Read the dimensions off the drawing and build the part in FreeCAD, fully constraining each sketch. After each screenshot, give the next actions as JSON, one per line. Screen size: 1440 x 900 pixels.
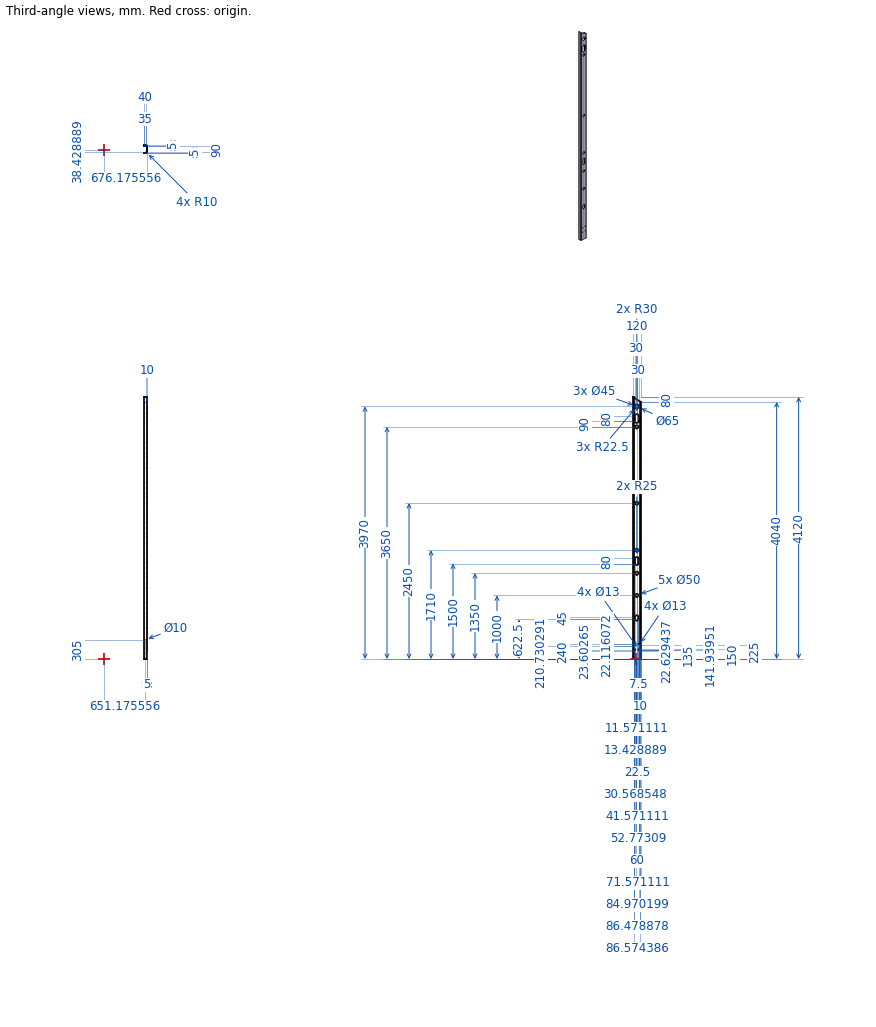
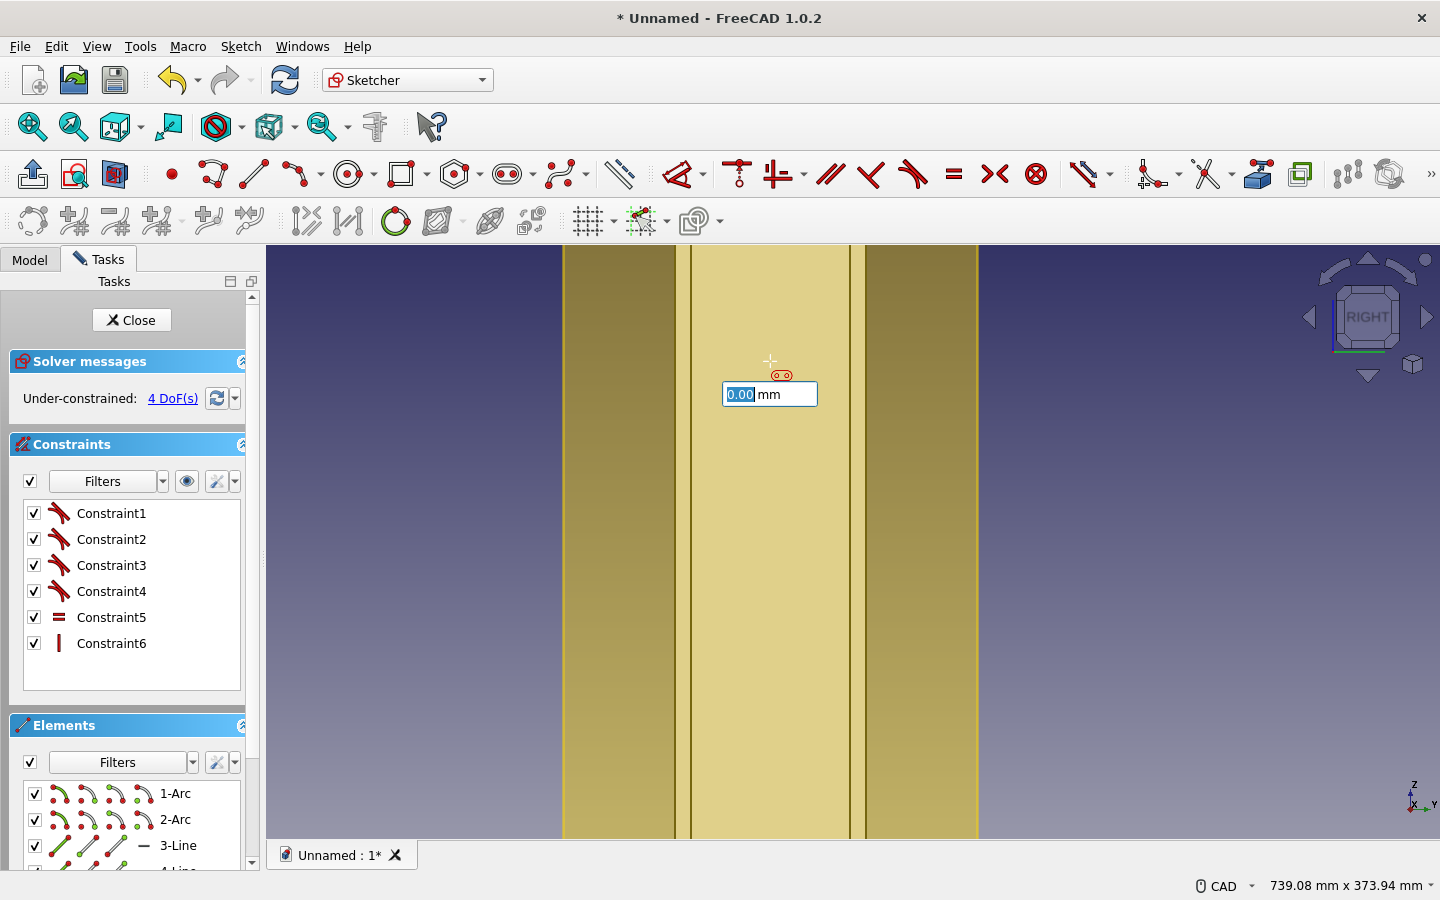
{"action": "scroll", "coordinate": [785, 366], "scroll_direction": "down", "scroll_amount": 14}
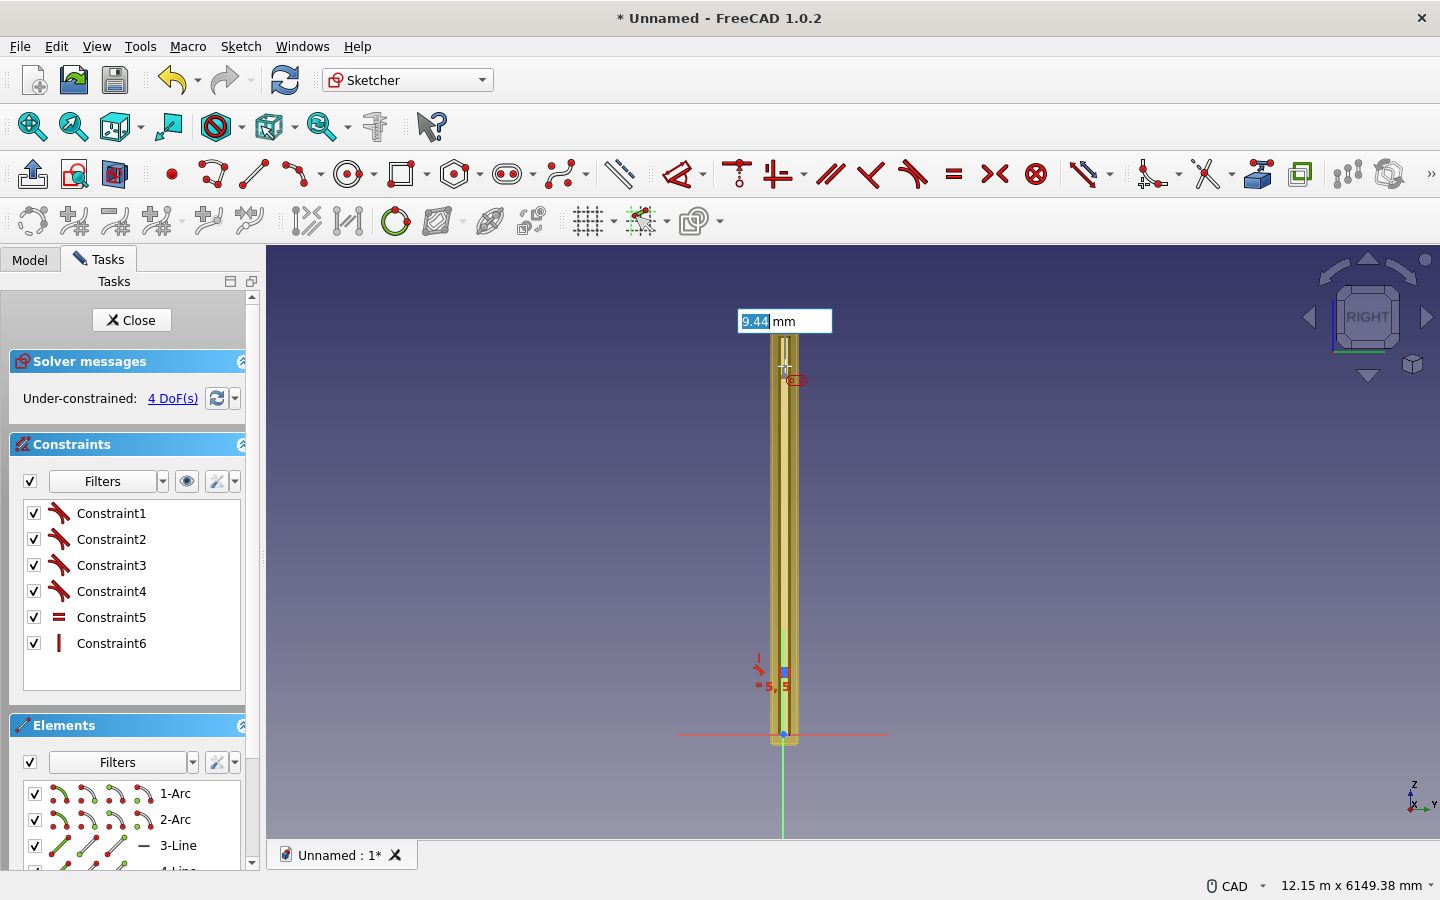
{"action": "scroll", "coordinate": [787, 370], "scroll_direction": "up", "scroll_amount": 9}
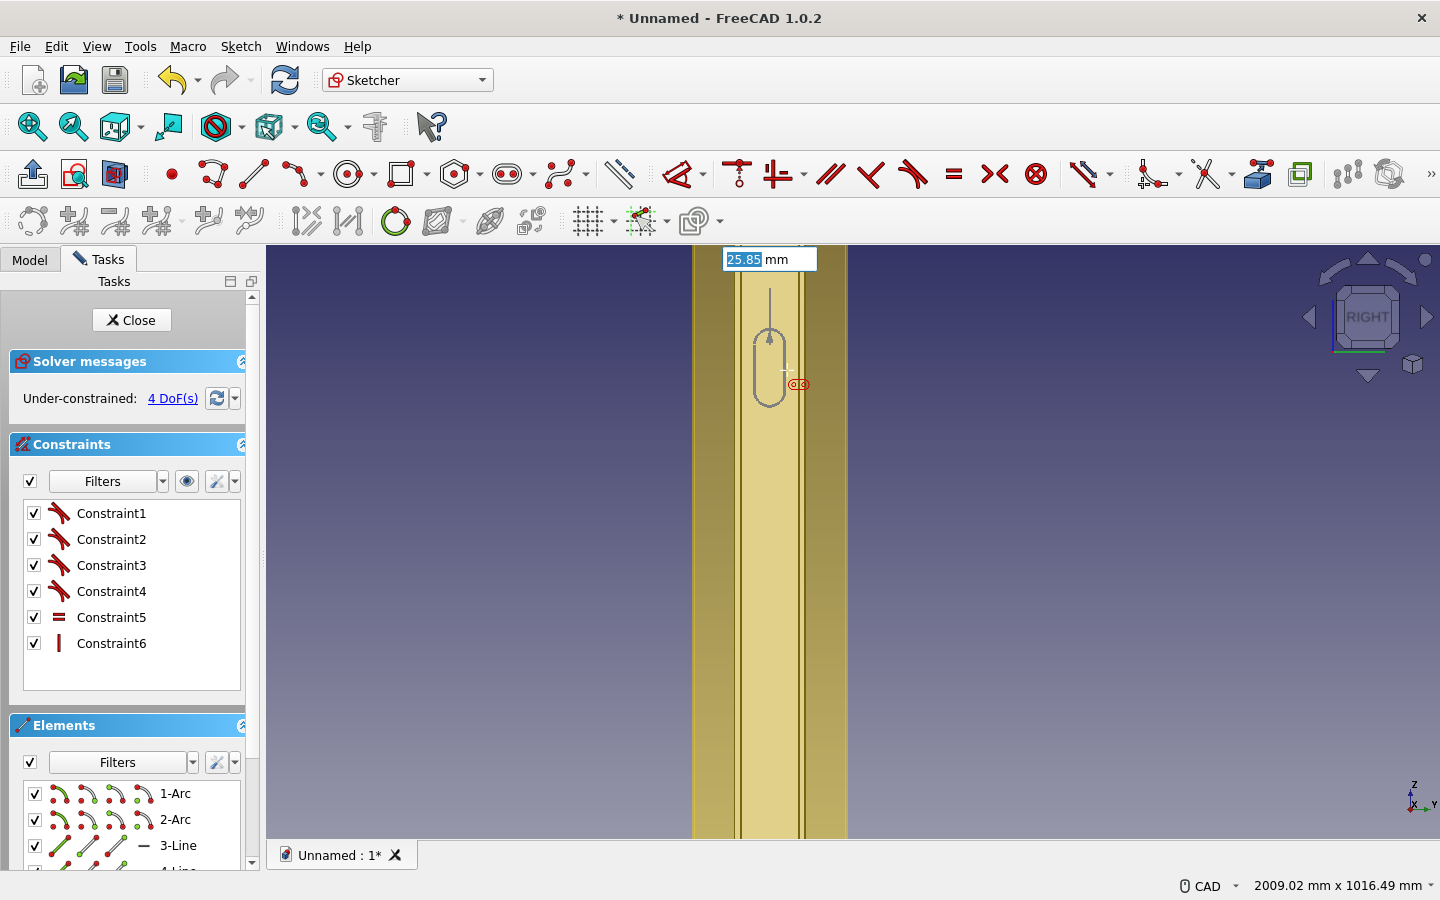
{"action": "left_click", "coordinate": [787, 367]}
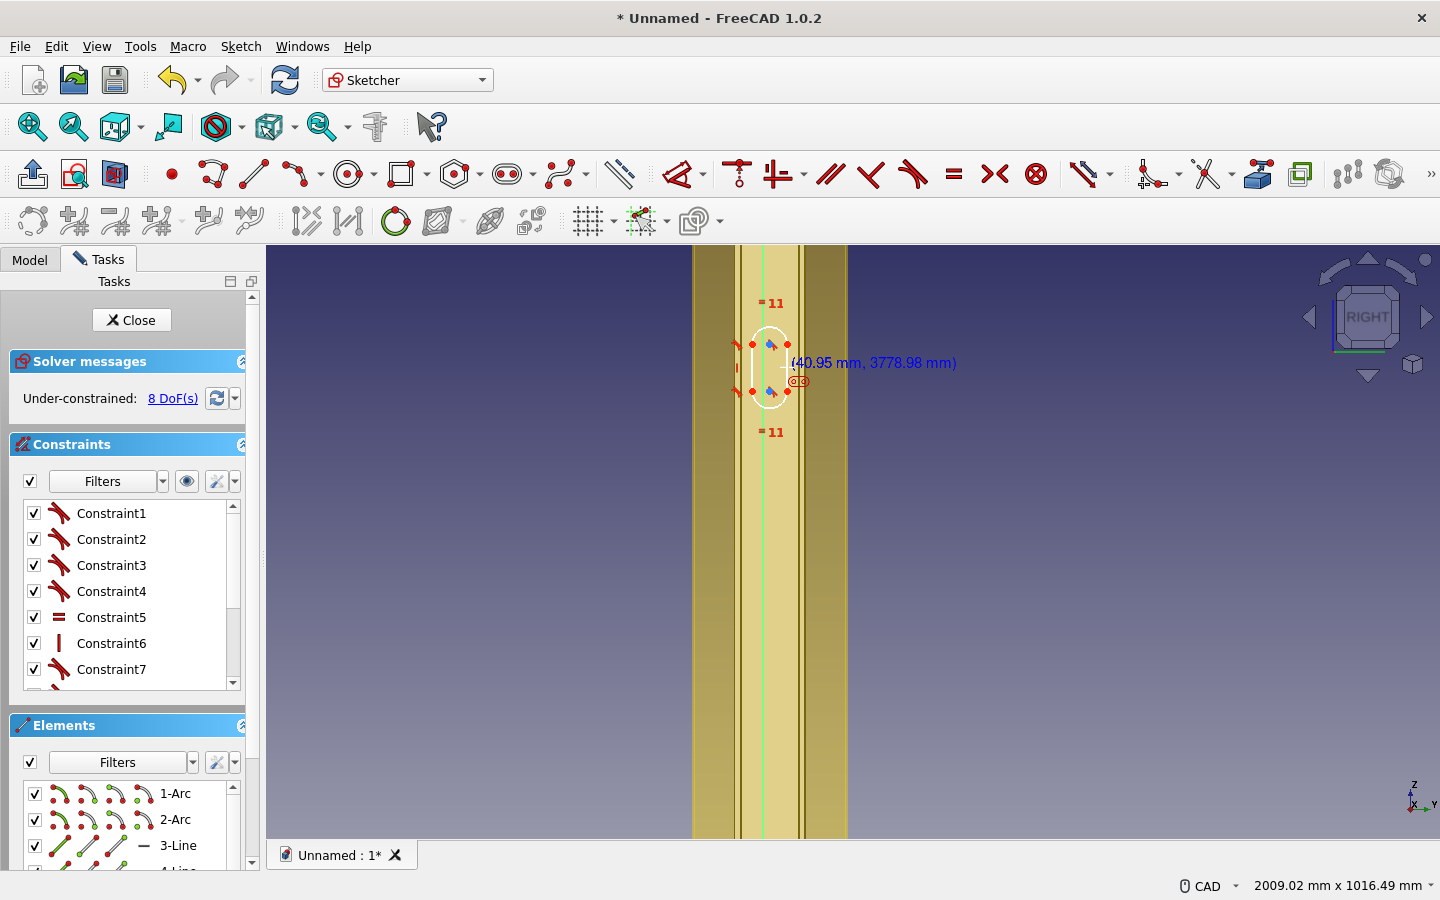
{"action": "key", "text": "g c"}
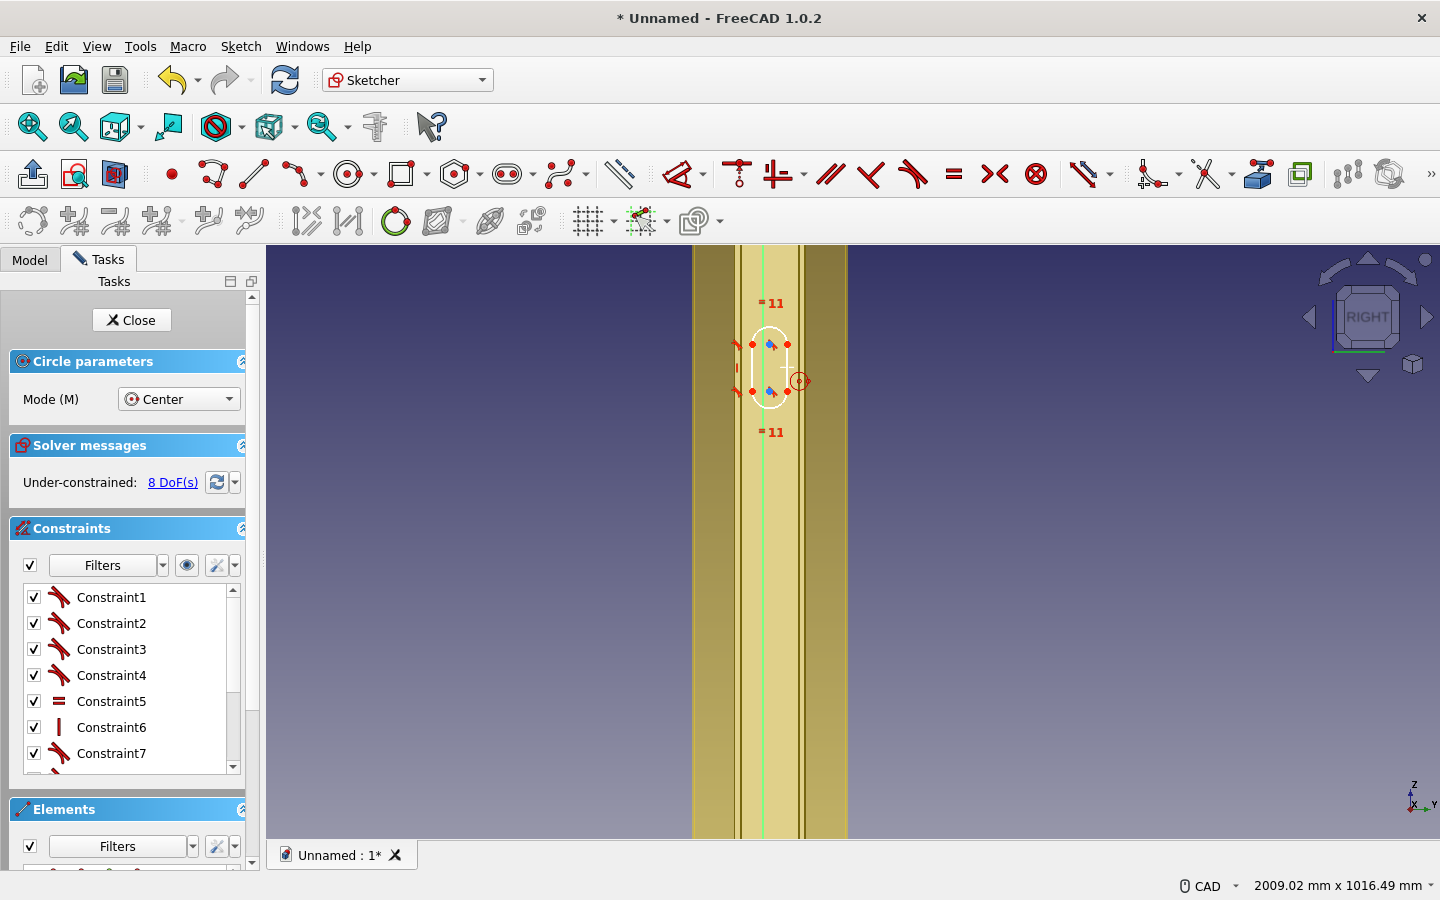
{"action": "scroll", "coordinate": [787, 370], "scroll_direction": "down", "scroll_amount": 9}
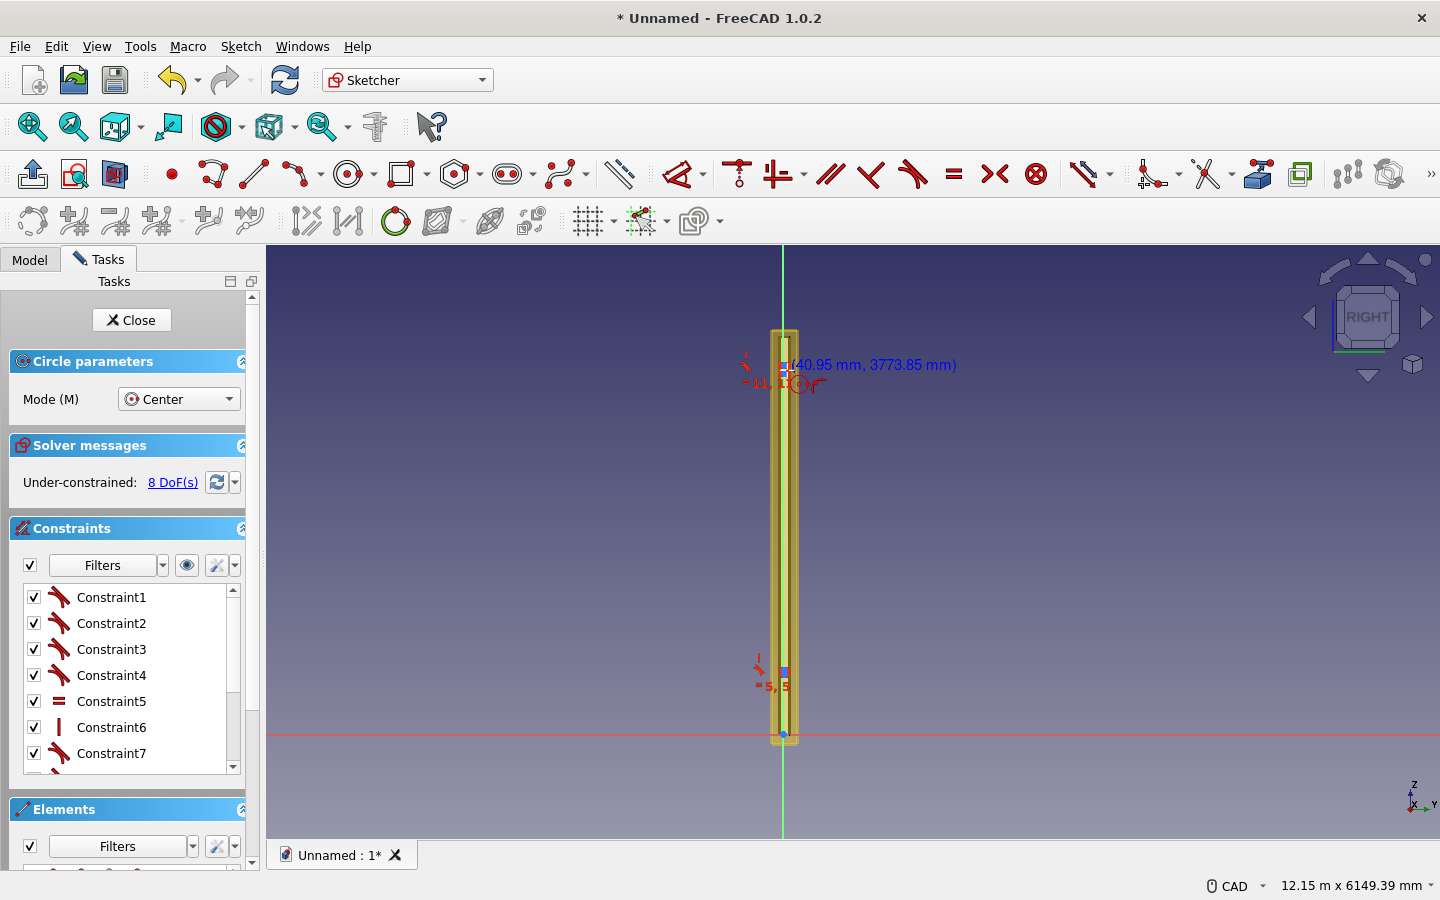
{"action": "scroll", "coordinate": [787, 713], "scroll_direction": "up", "scroll_amount": 18}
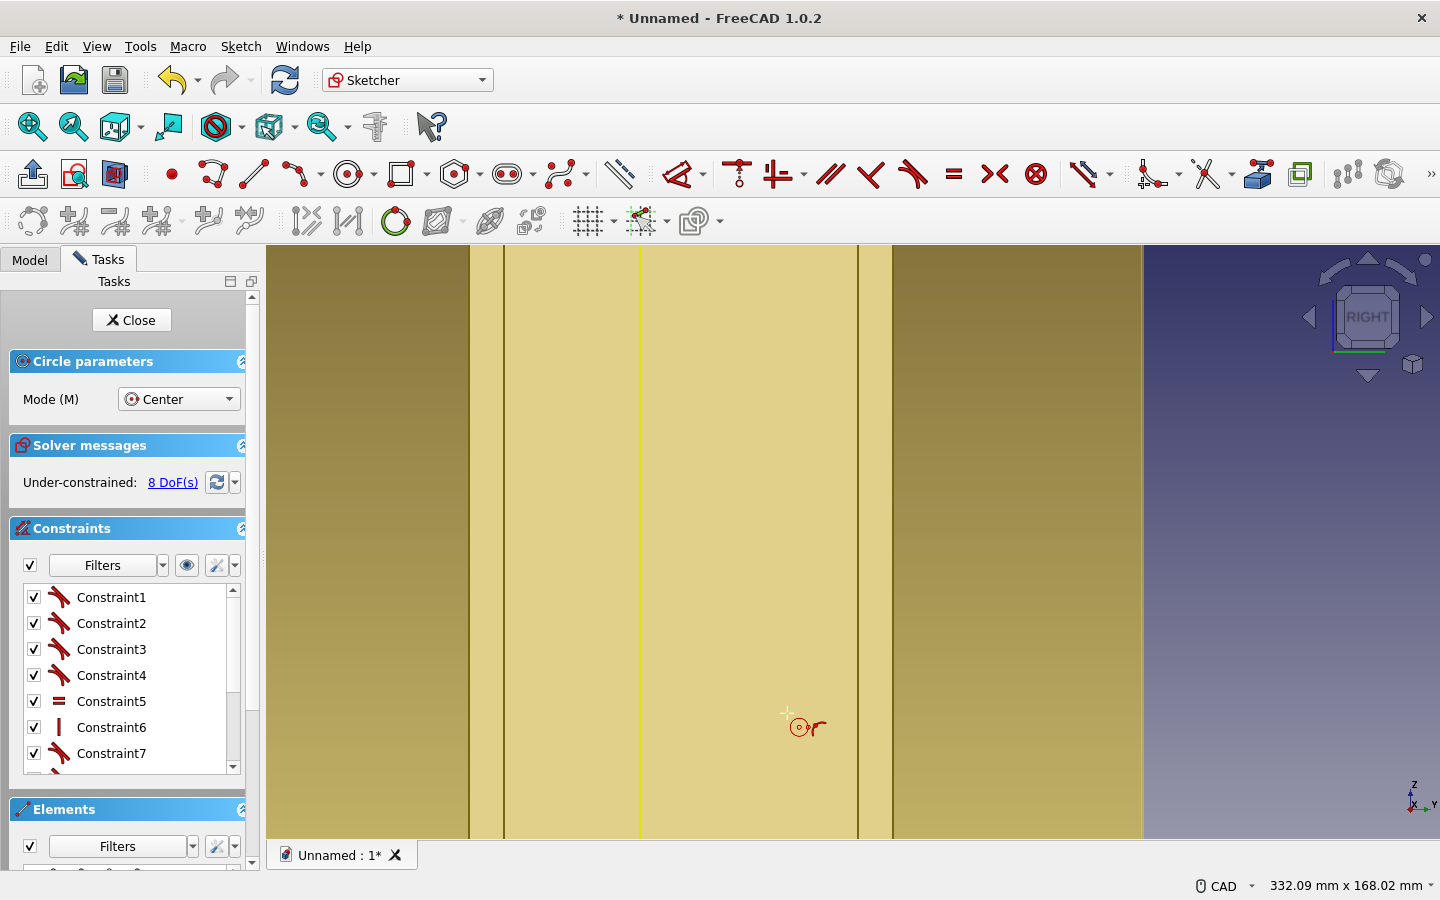
{"action": "scroll", "coordinate": [788, 753], "scroll_direction": "down", "scroll_amount": 17}